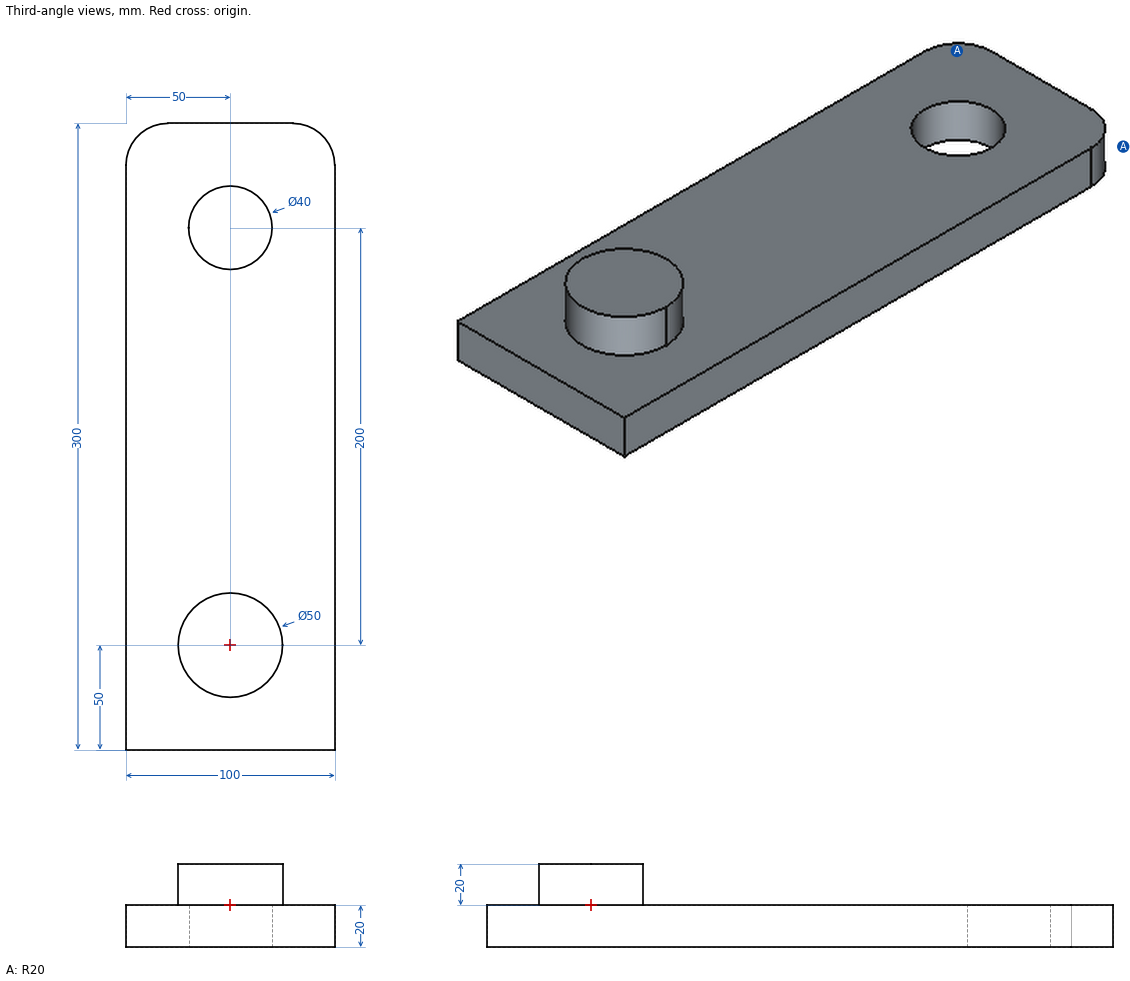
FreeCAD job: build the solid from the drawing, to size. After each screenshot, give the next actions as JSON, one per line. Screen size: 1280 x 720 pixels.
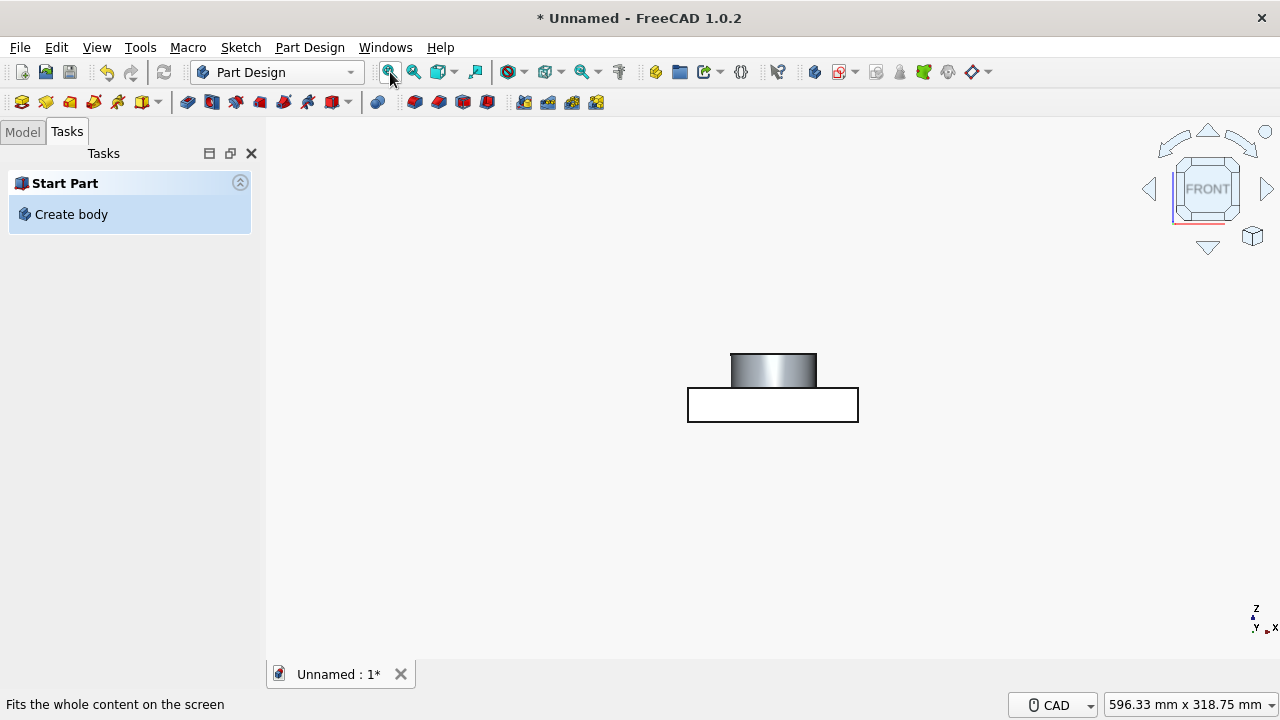
{"action": "left_click", "coordinate": [390, 72]}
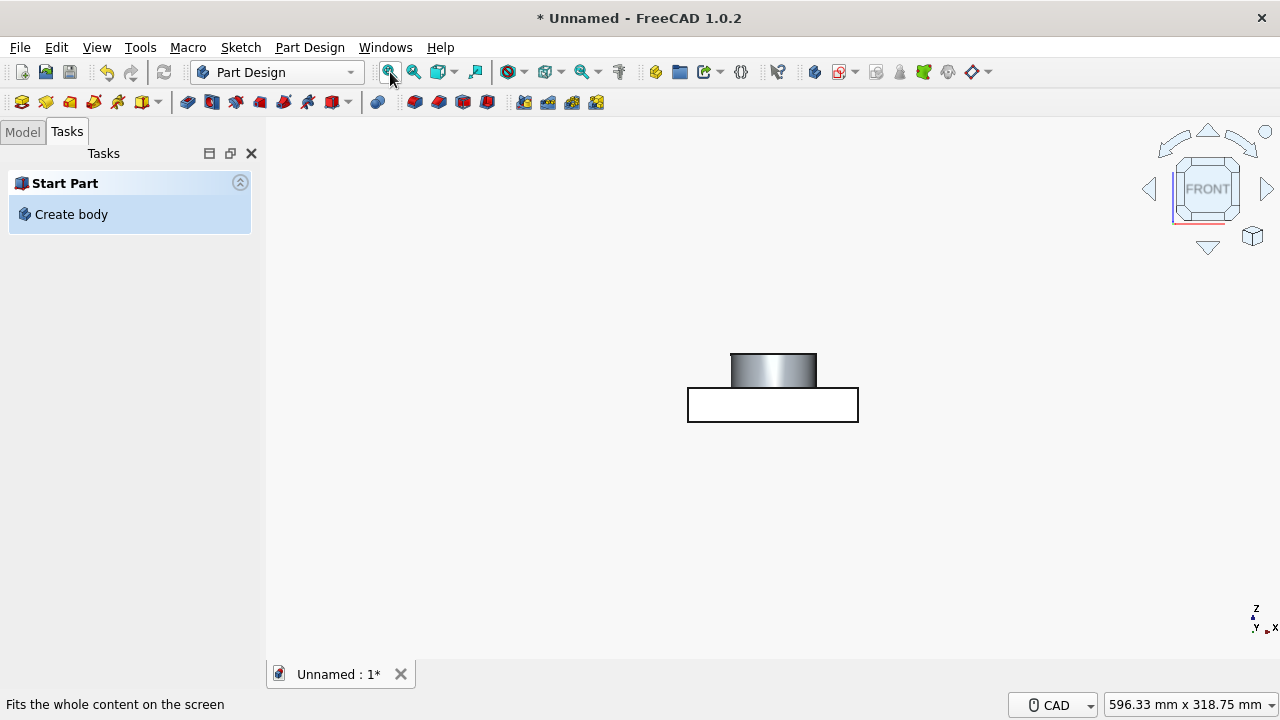
{"action": "key", "text": "3"}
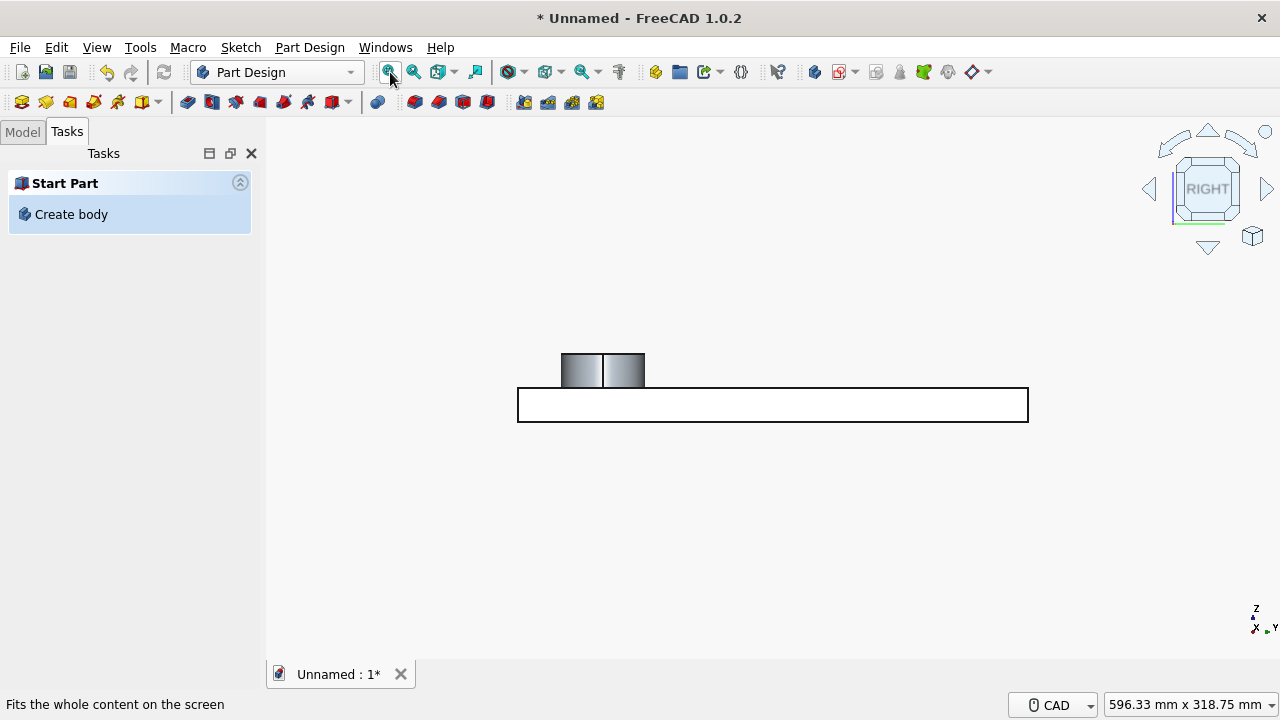
{"action": "left_click", "coordinate": [1028, 404]}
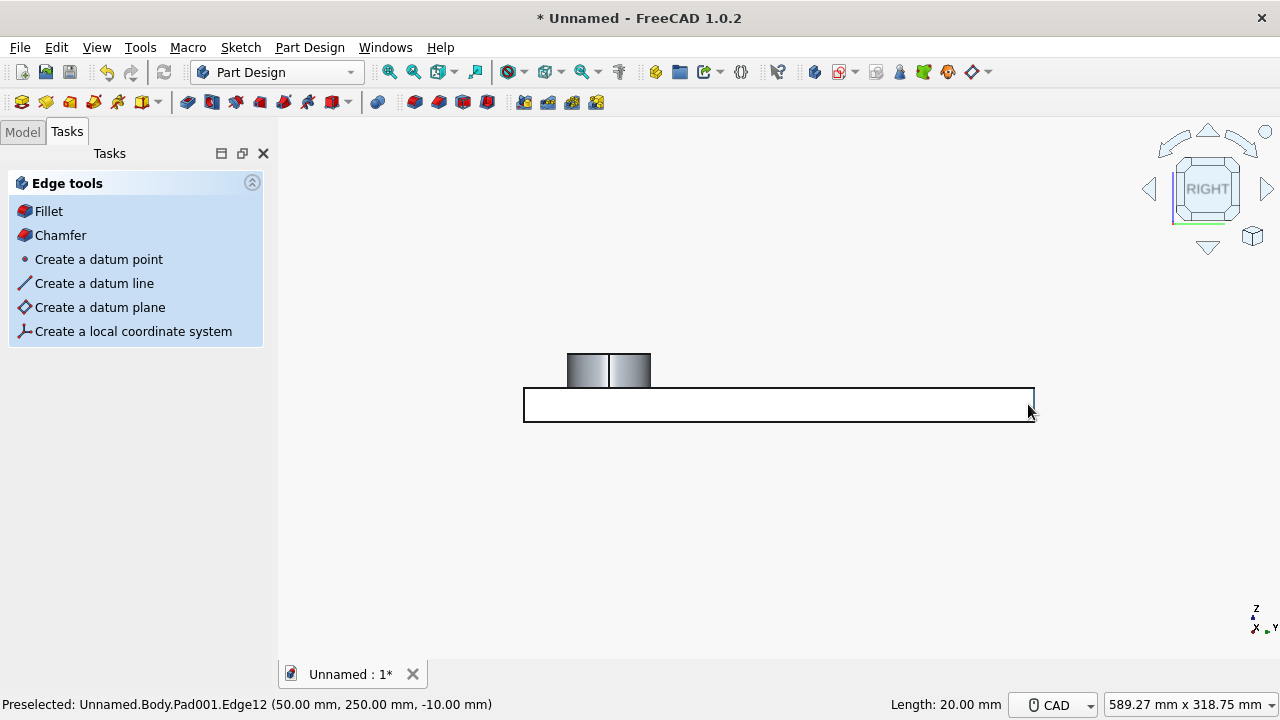
{"action": "key", "text": "5"}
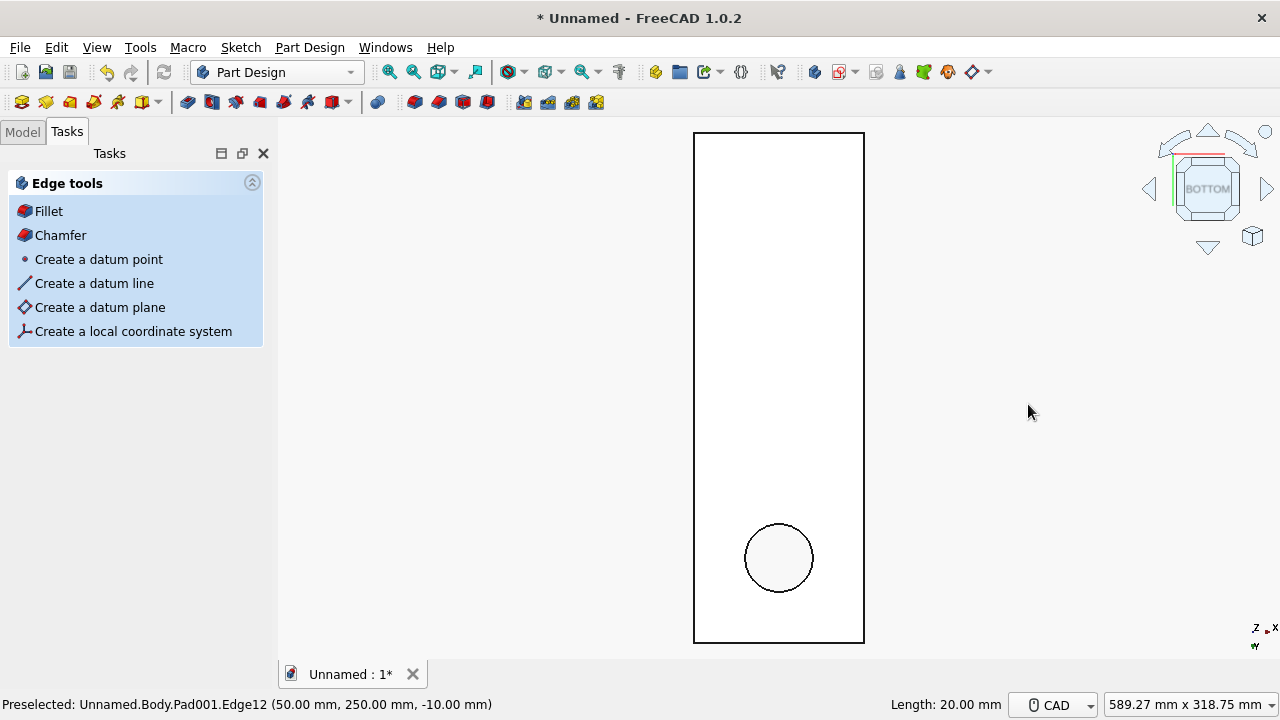
{"action": "key", "text": "4"}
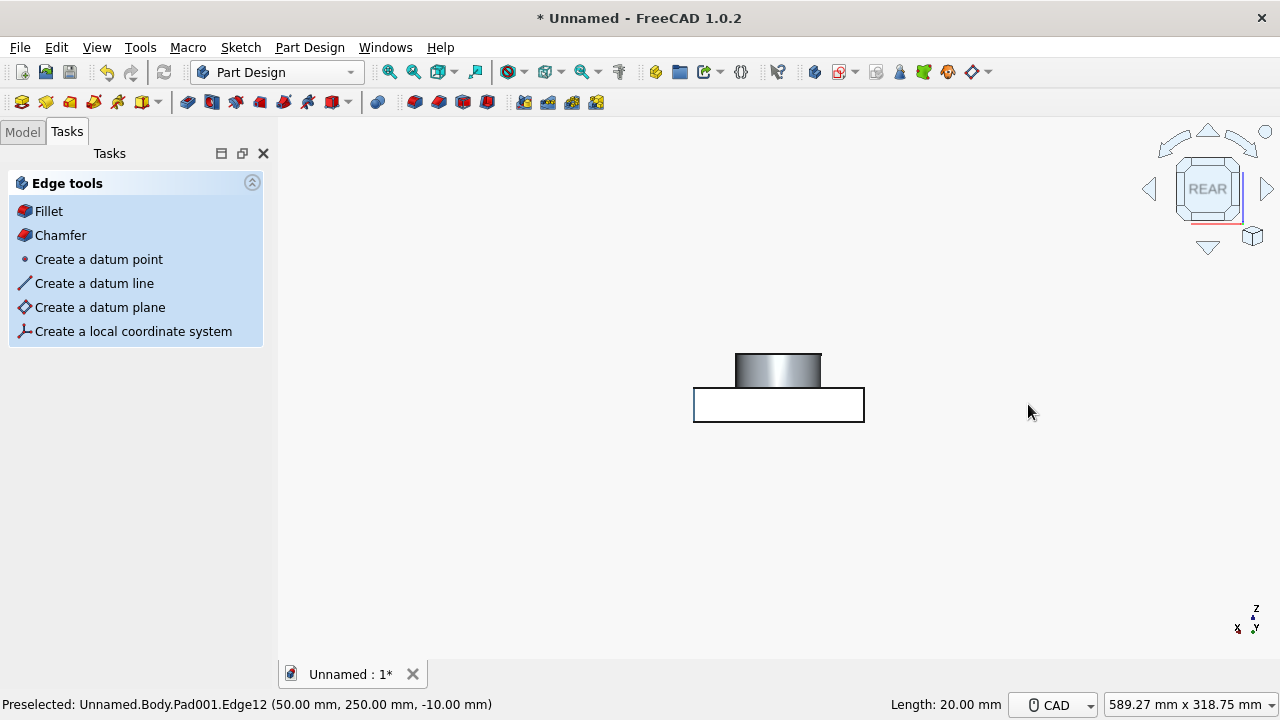
{"action": "left_click", "coordinate": [390, 72]}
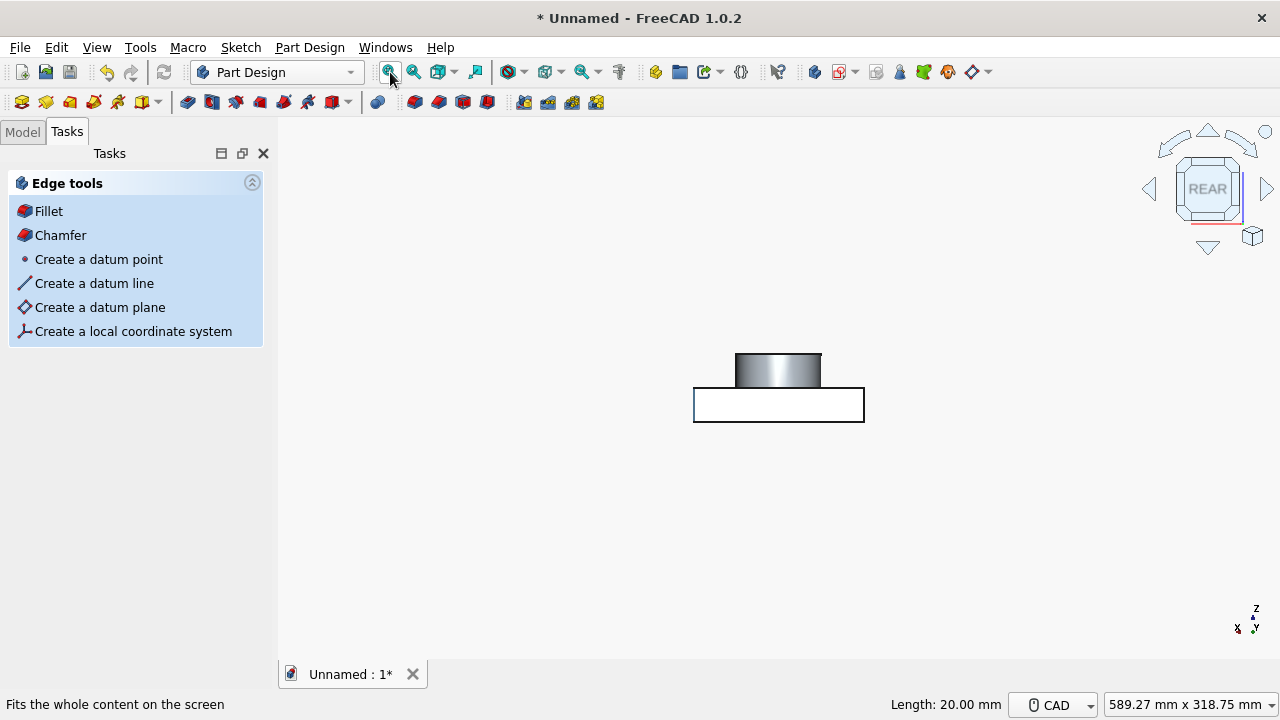
{"action": "left_click", "coordinate": [864, 404], "text": "ctrl"}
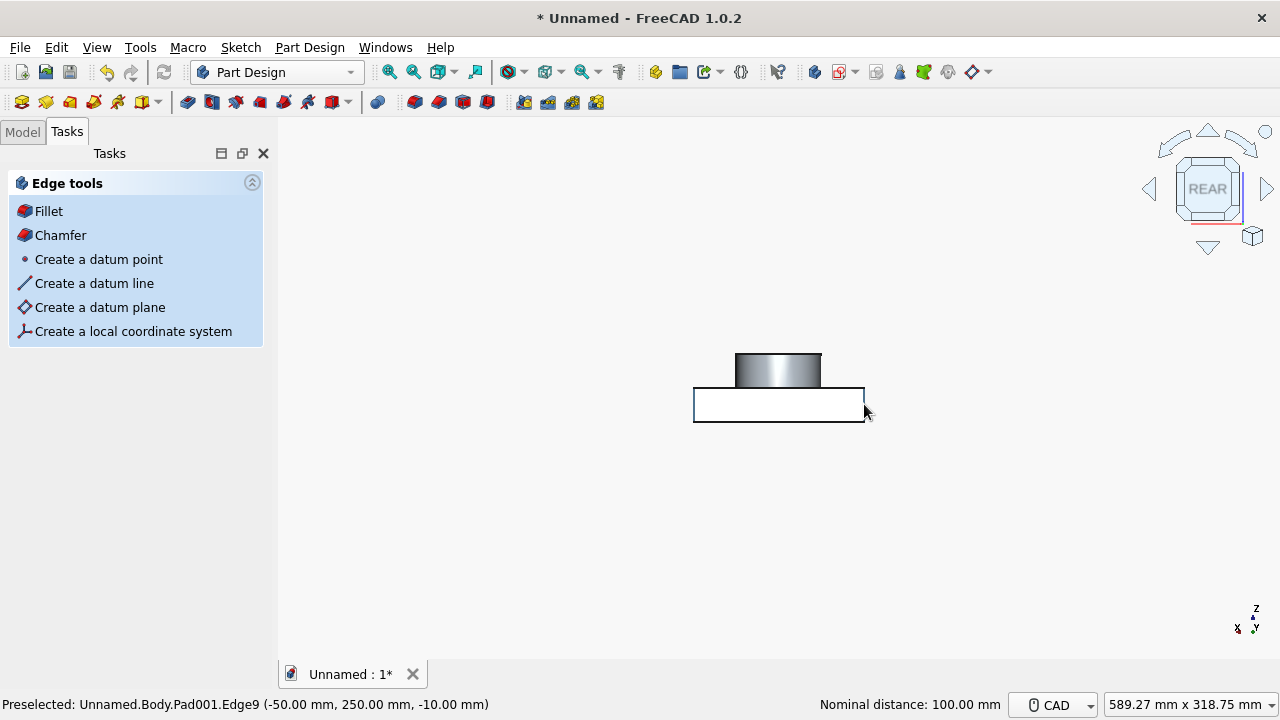
{"action": "left_click", "coordinate": [416, 102]}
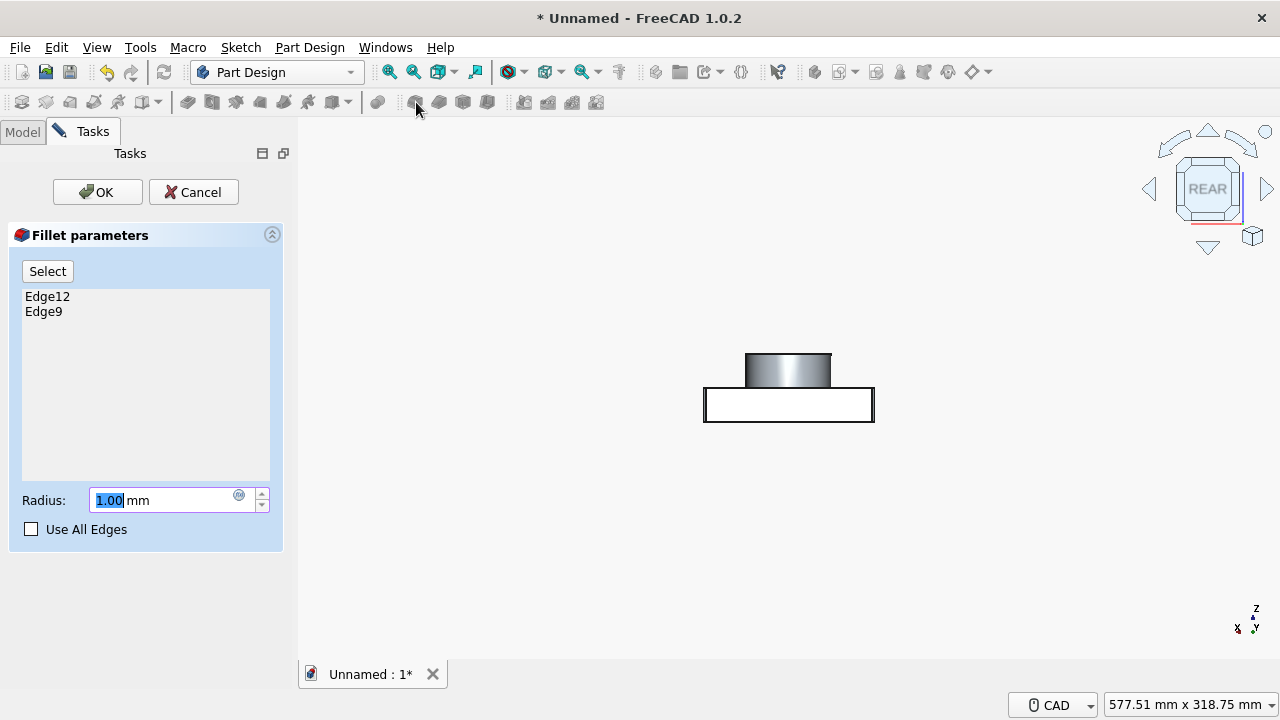
{"action": "type", "text": "20"}
{"action": "key", "text": "Tab"}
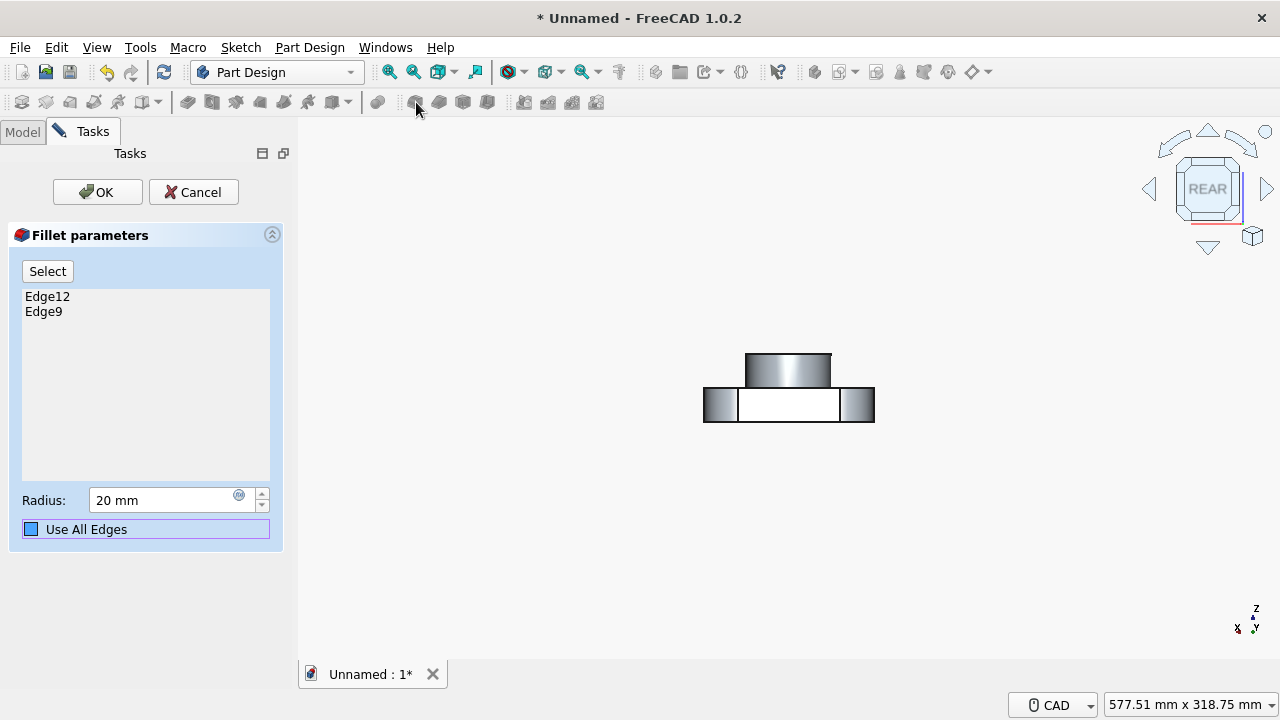
{"action": "left_click", "coordinate": [98, 192]}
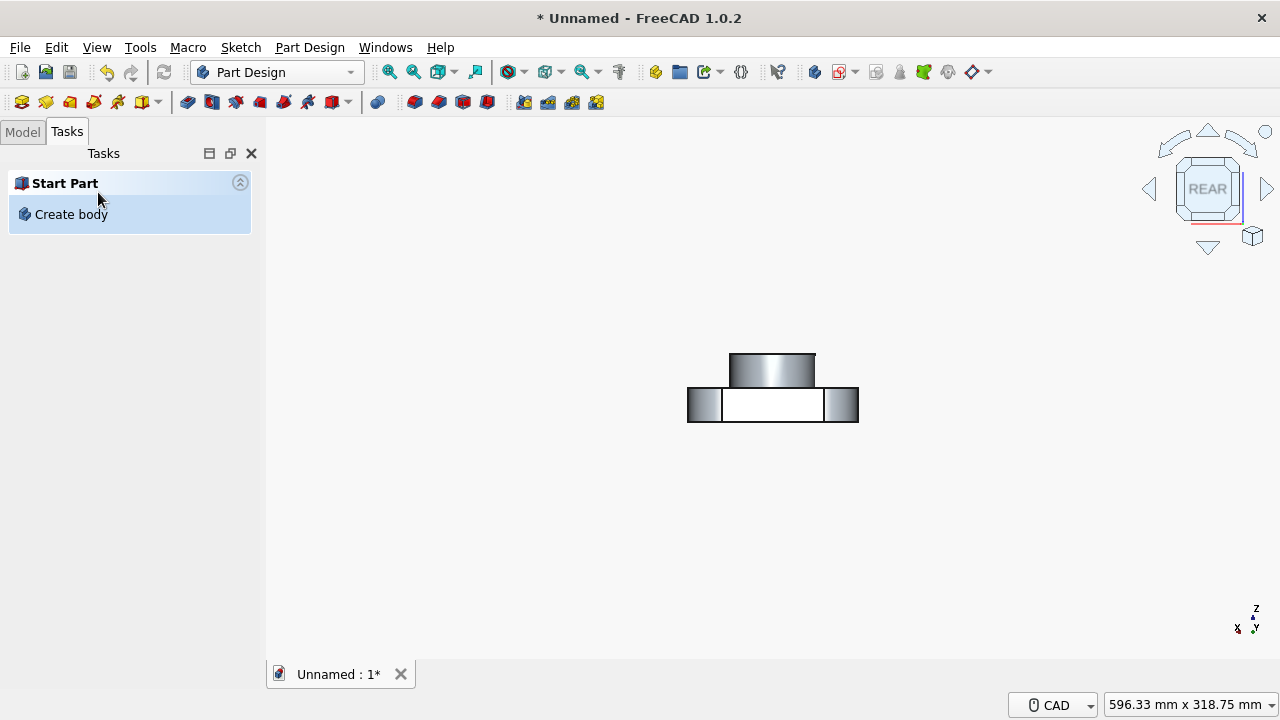
{"action": "key", "text": "0"}